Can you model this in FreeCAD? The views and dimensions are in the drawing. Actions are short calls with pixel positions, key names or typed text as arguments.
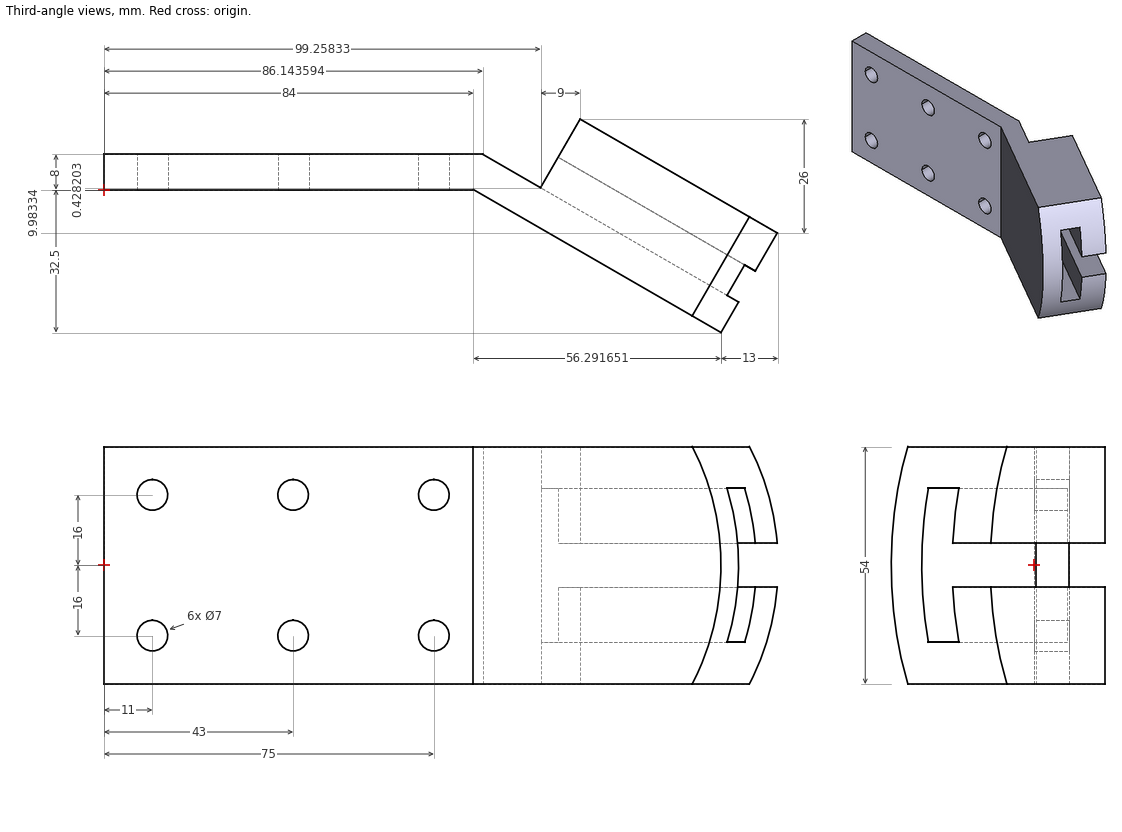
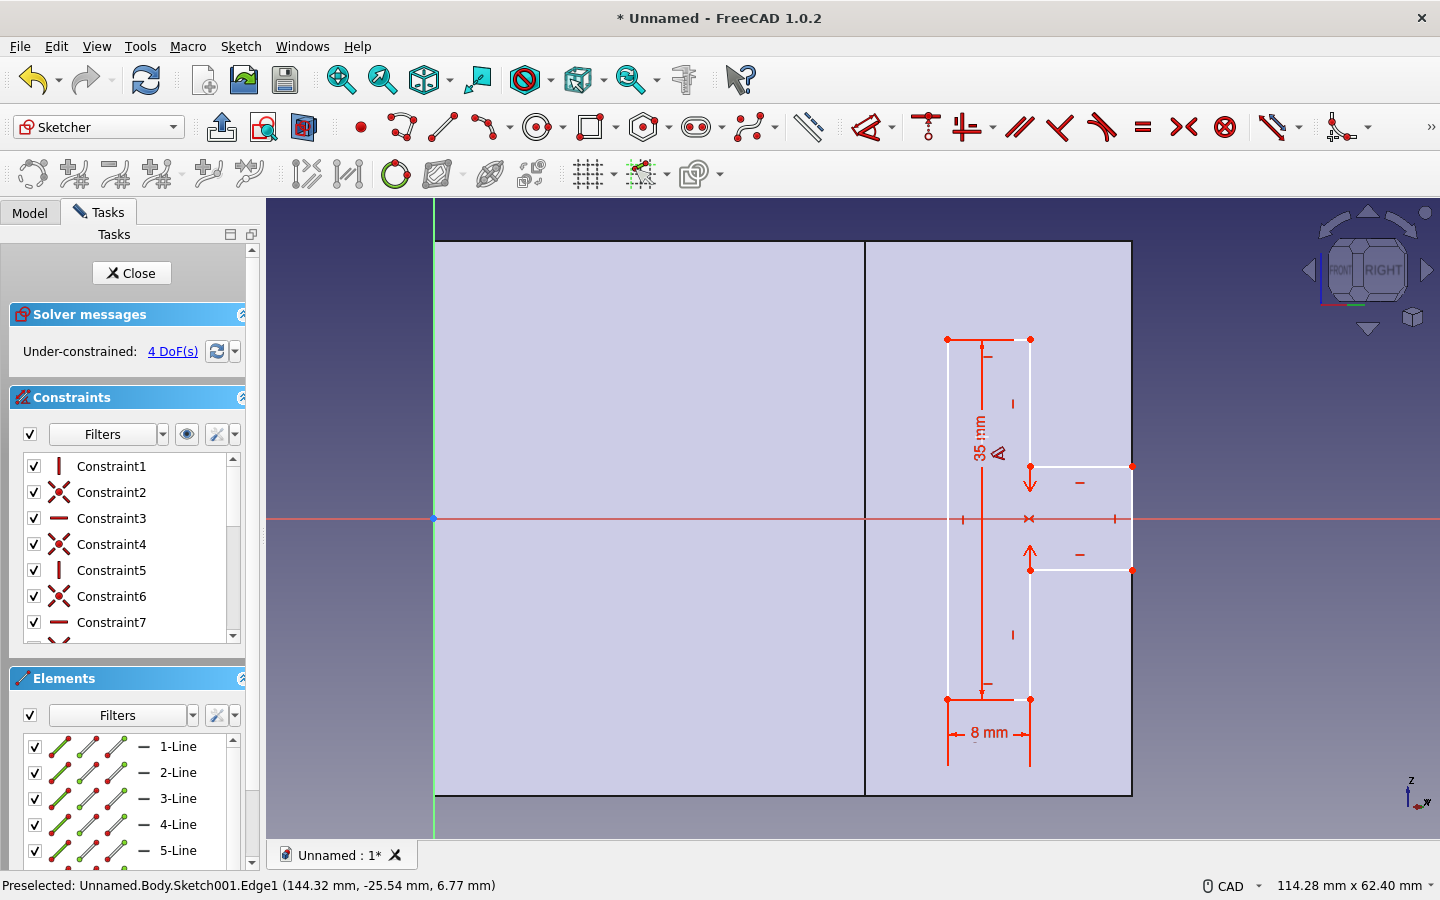
click(1061, 570)
click(1081, 604)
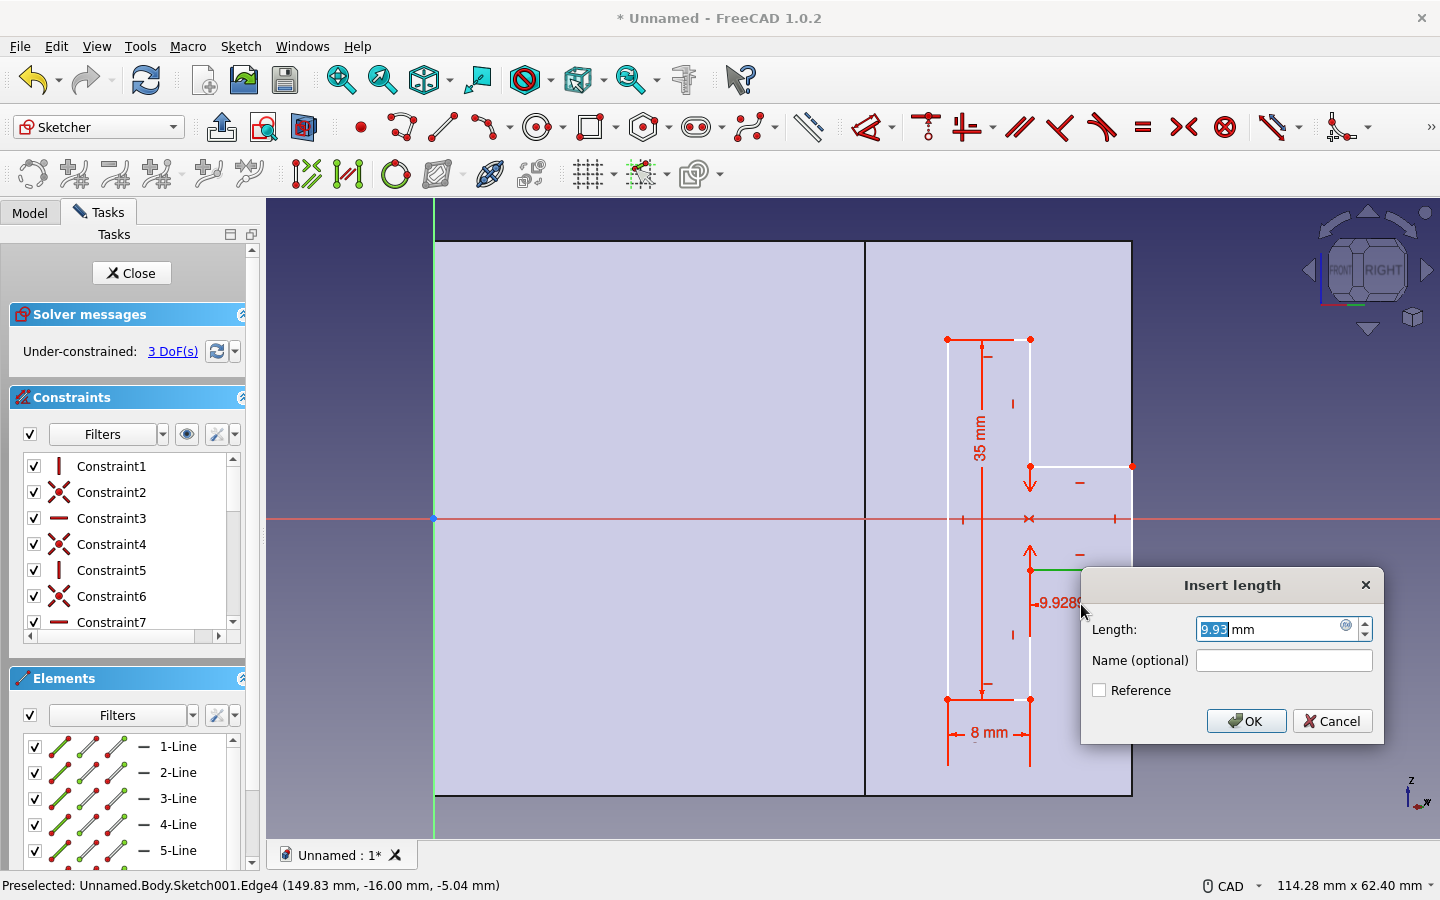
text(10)
key(Return)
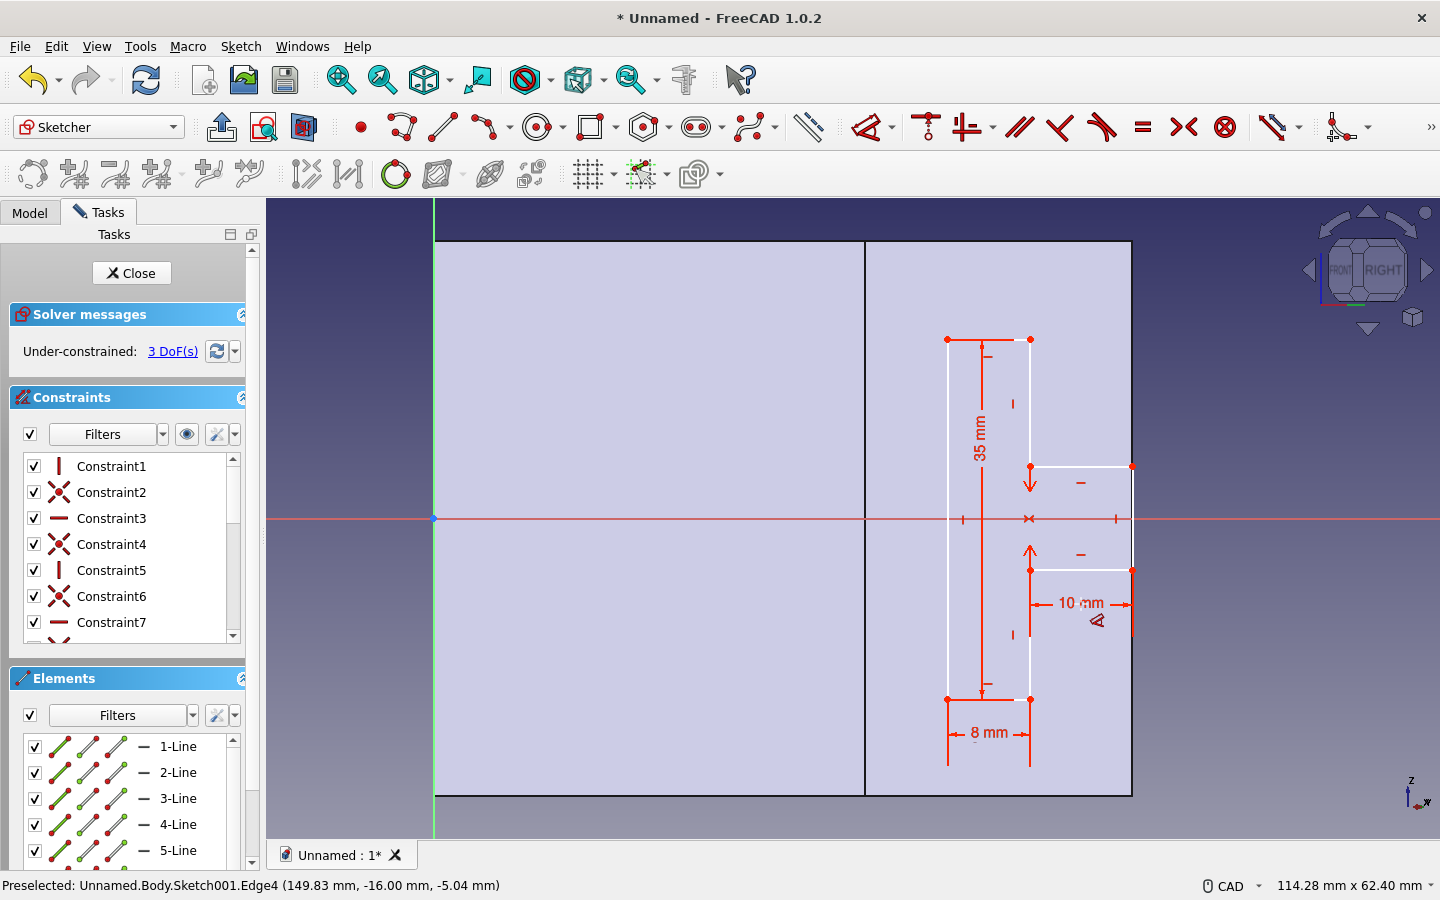
click(1133, 539)
click(1167, 495)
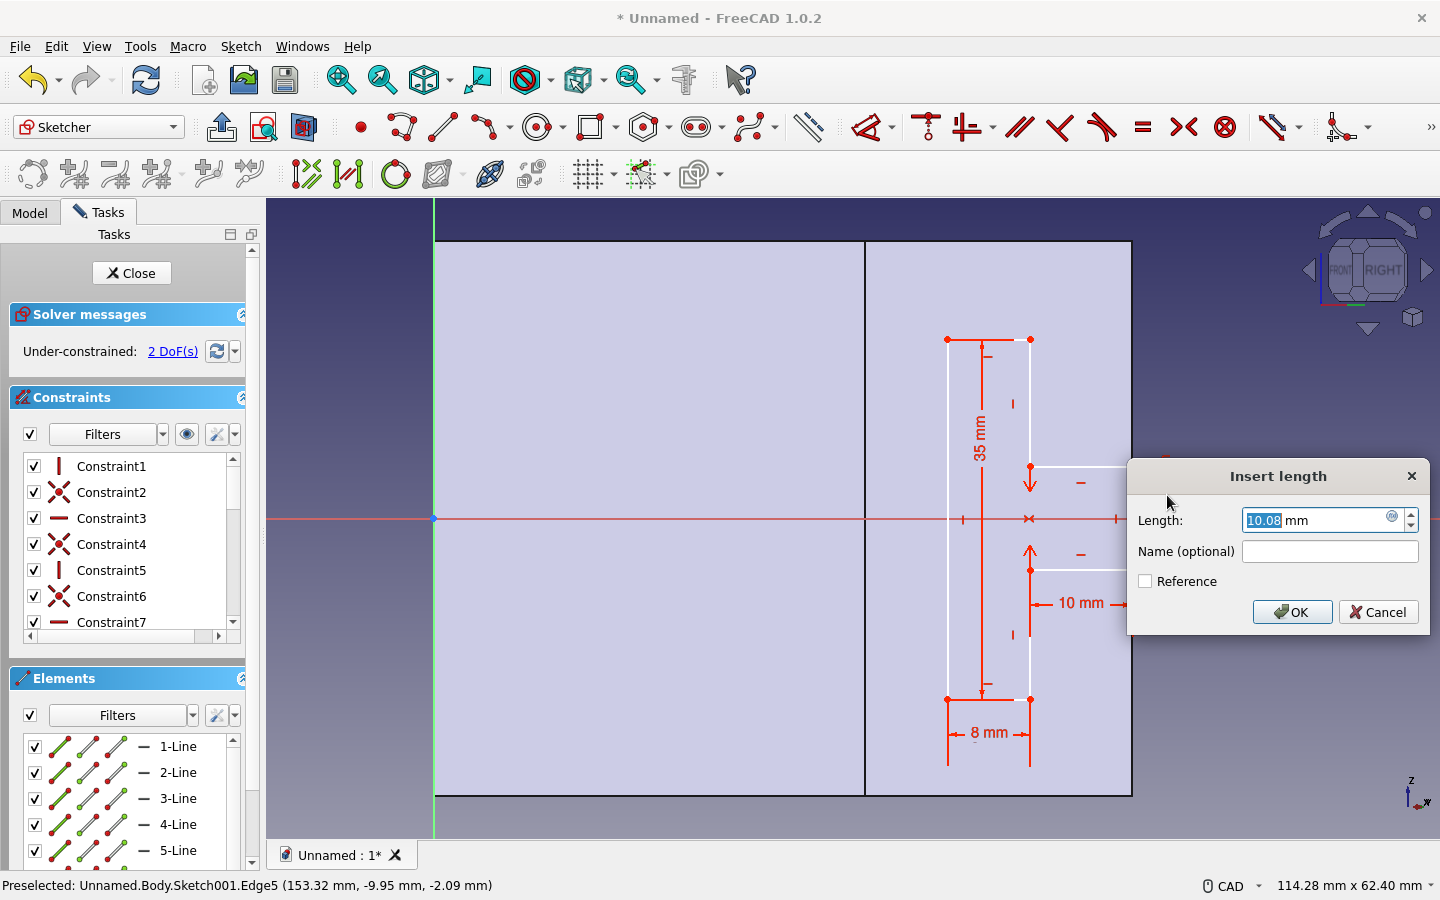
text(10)
key(Return)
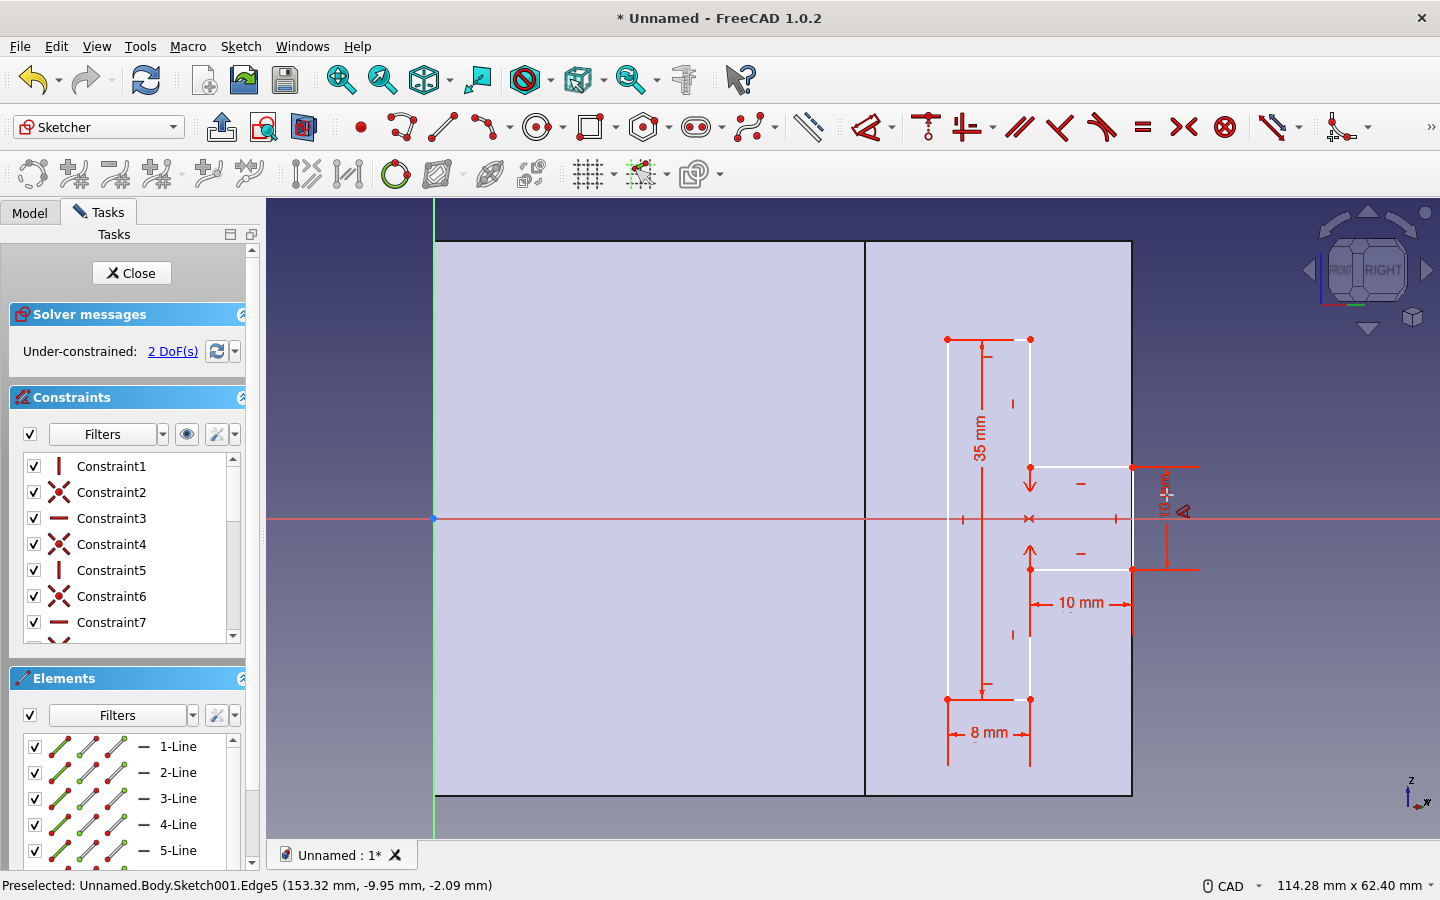
click(1030, 661)
click(1064, 635)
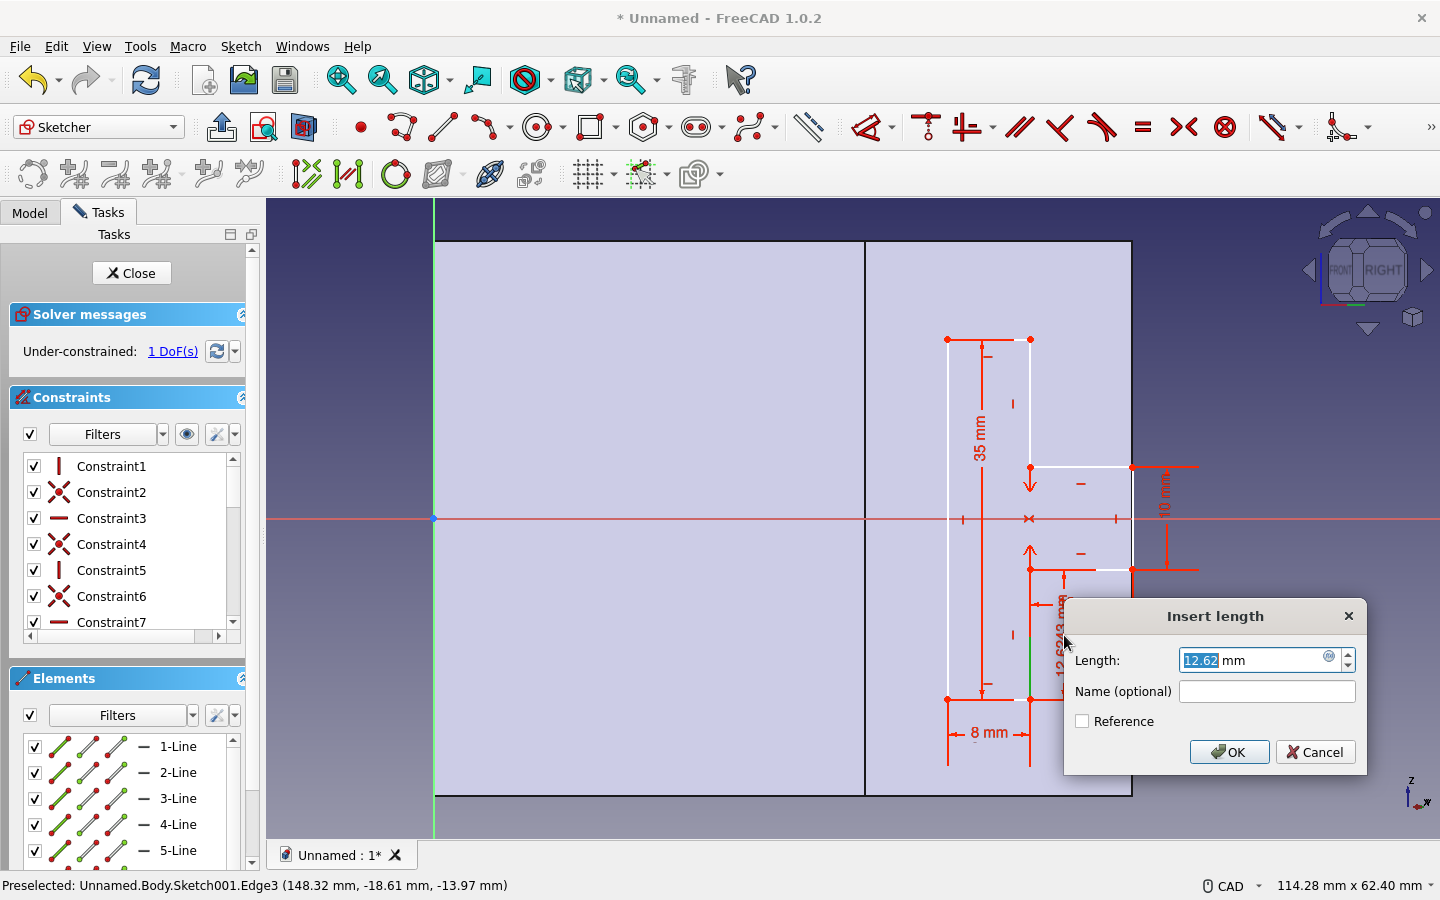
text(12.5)
key(Return)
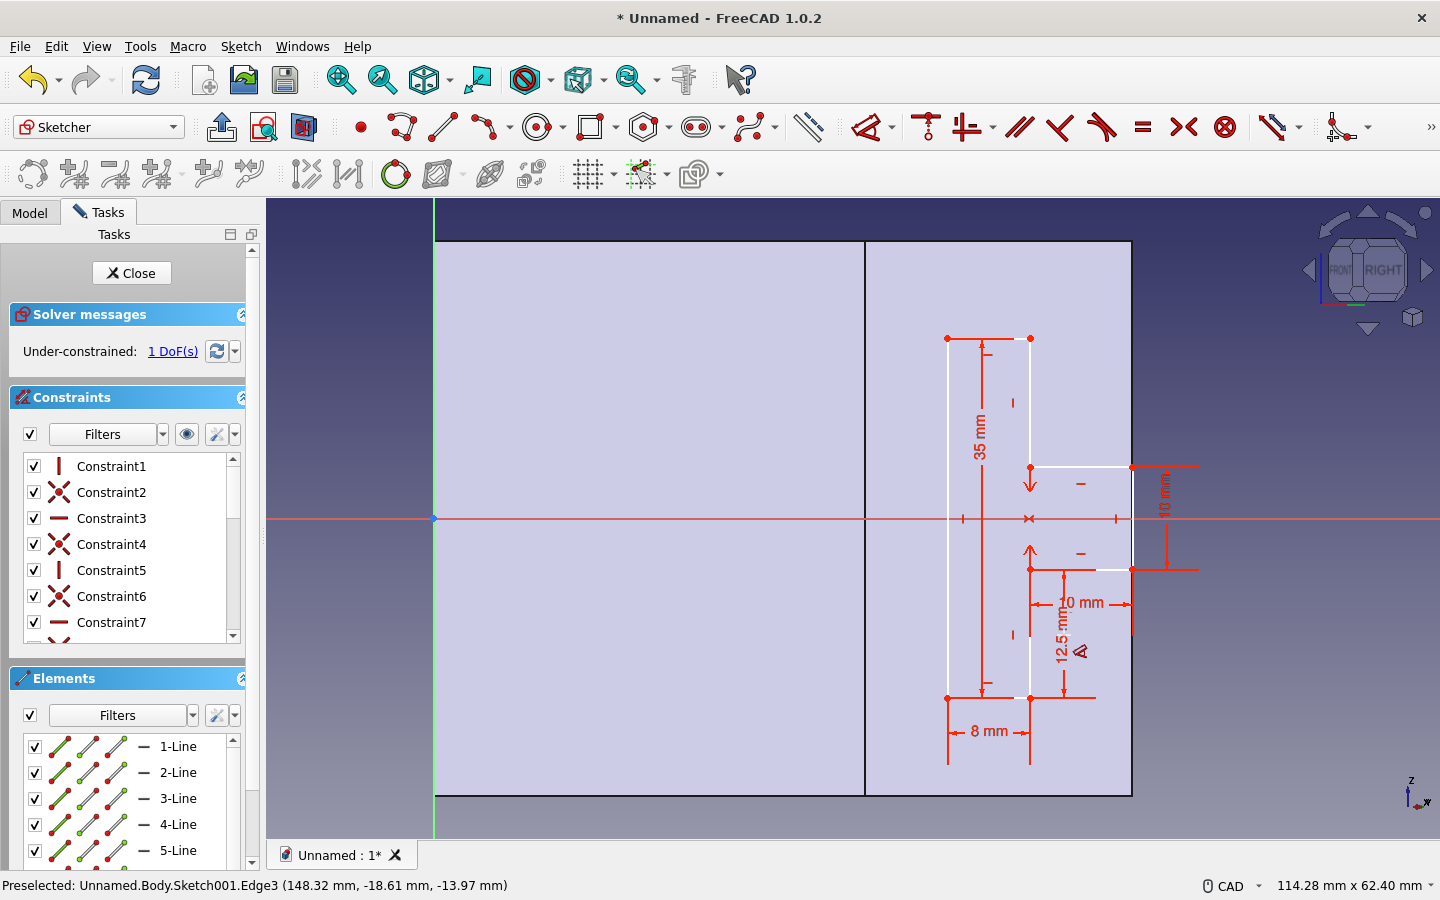
click(948, 339)
click(691, 305)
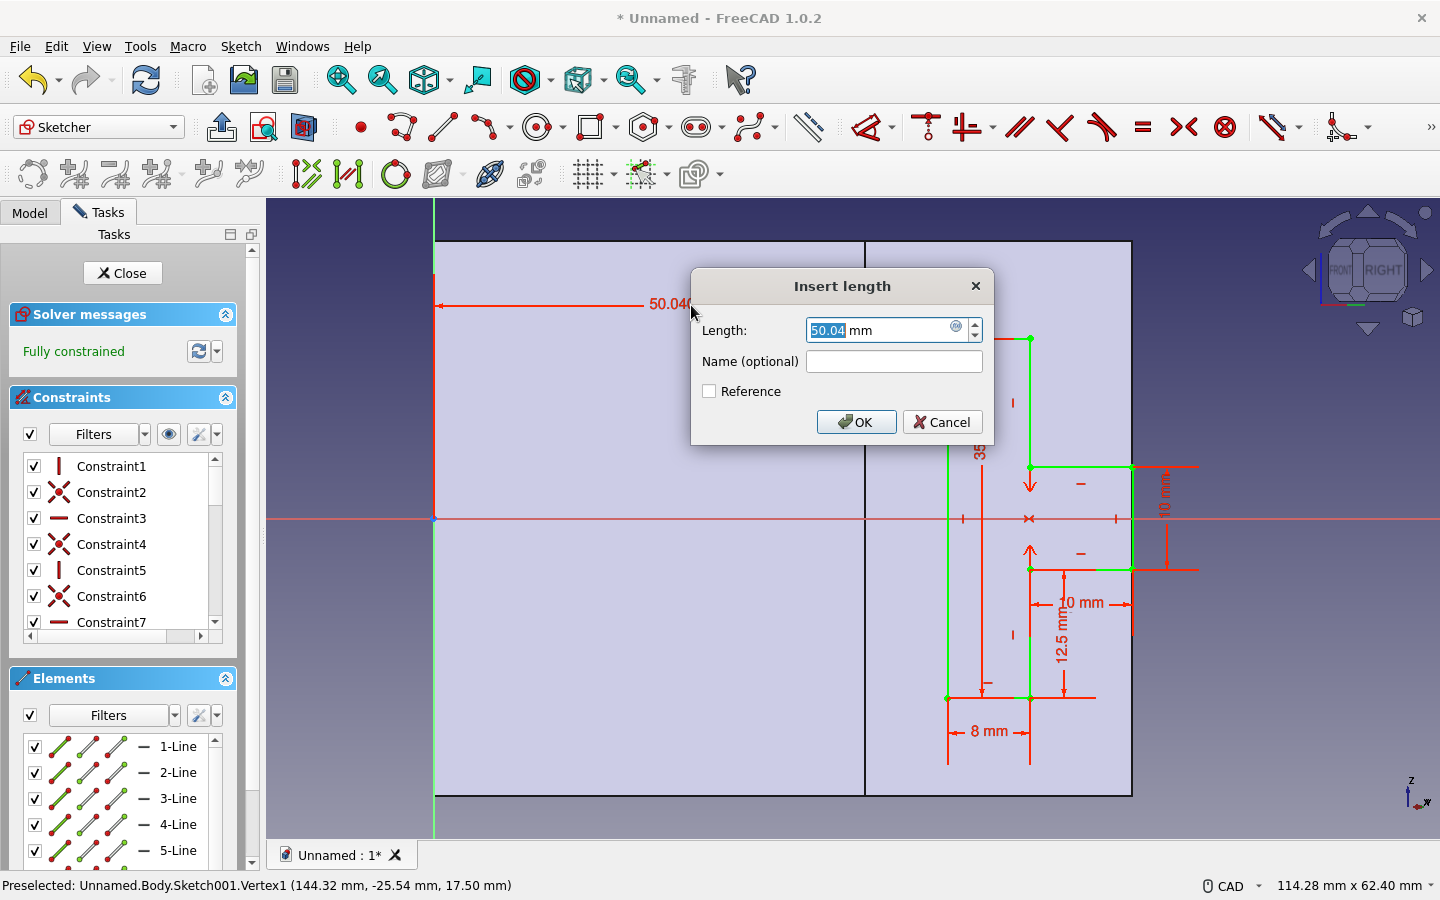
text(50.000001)
key(Return)
key(Escape)